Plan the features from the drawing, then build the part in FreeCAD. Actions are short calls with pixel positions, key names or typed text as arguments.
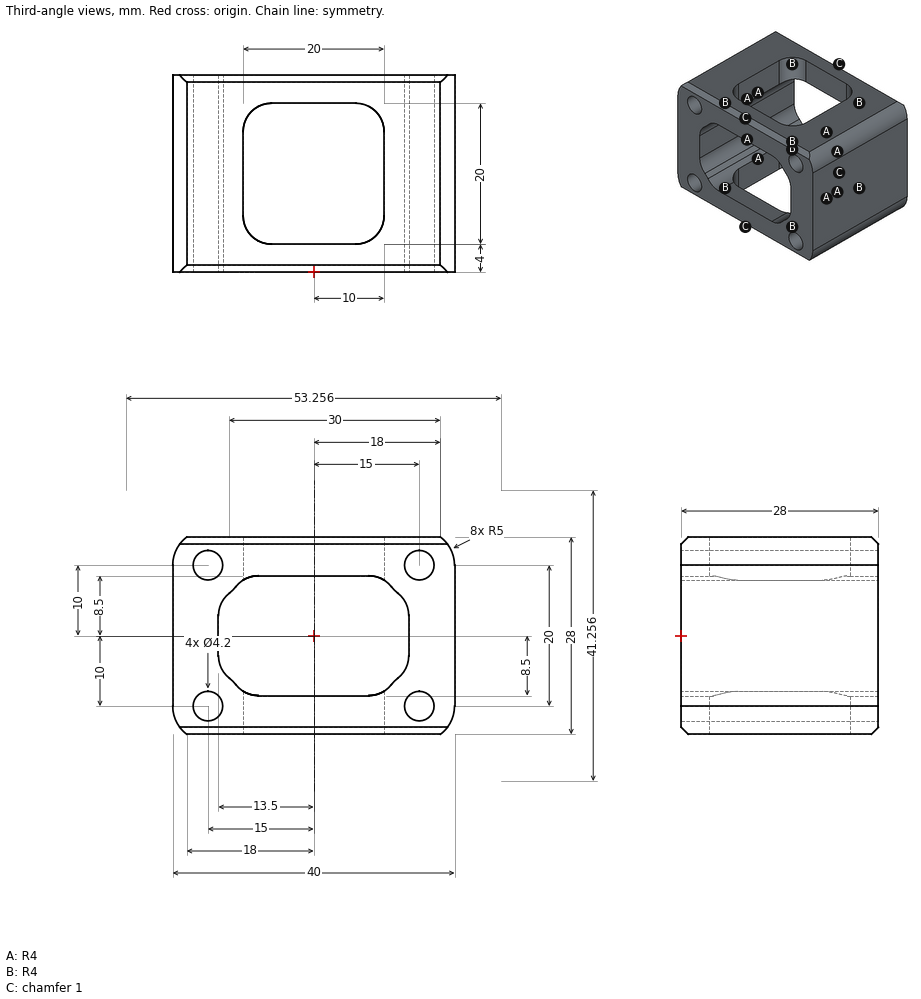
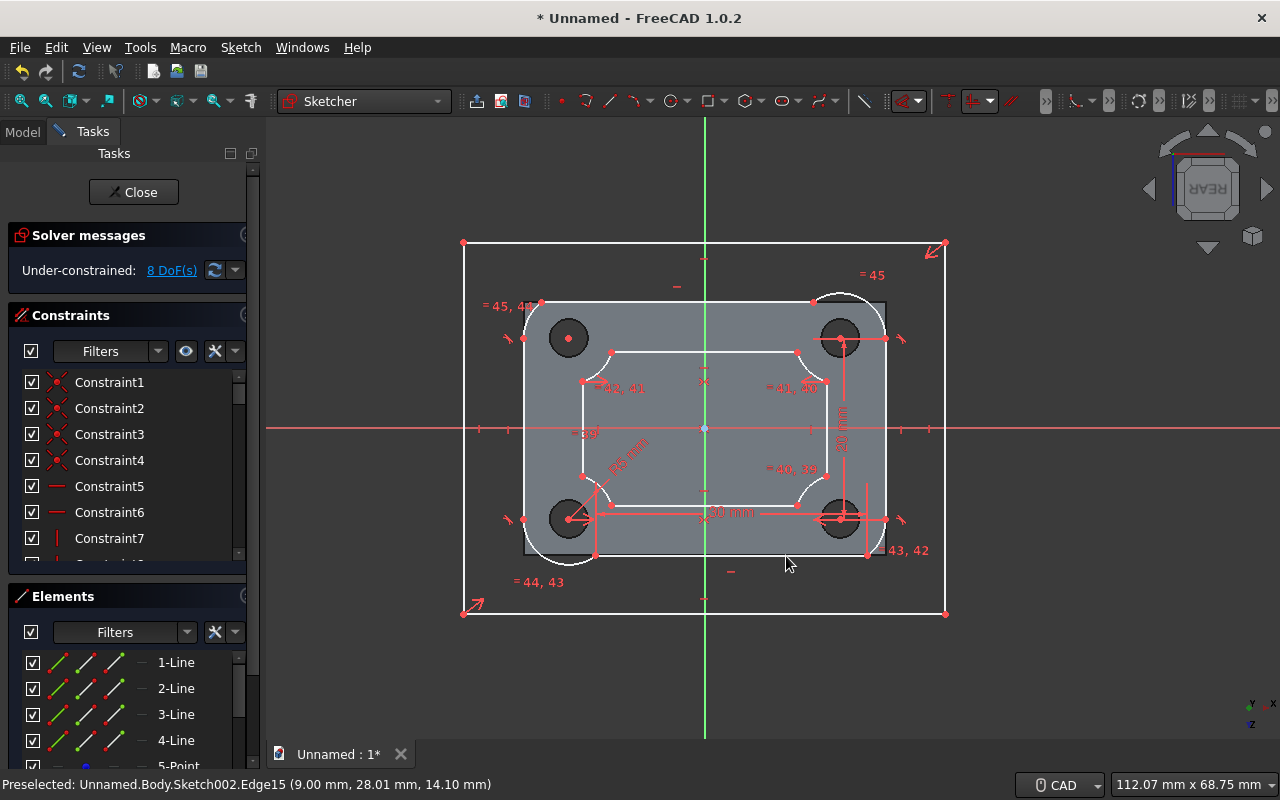
click(886, 339)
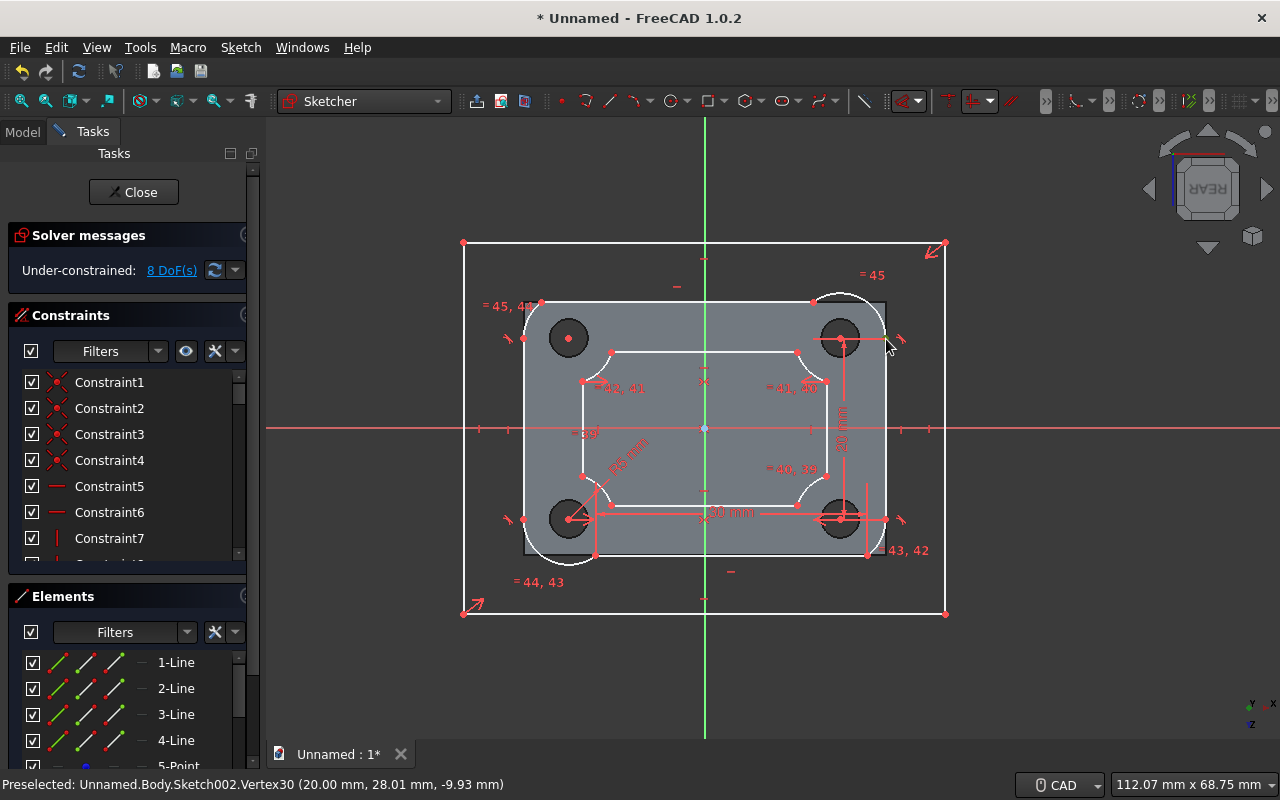
key(i)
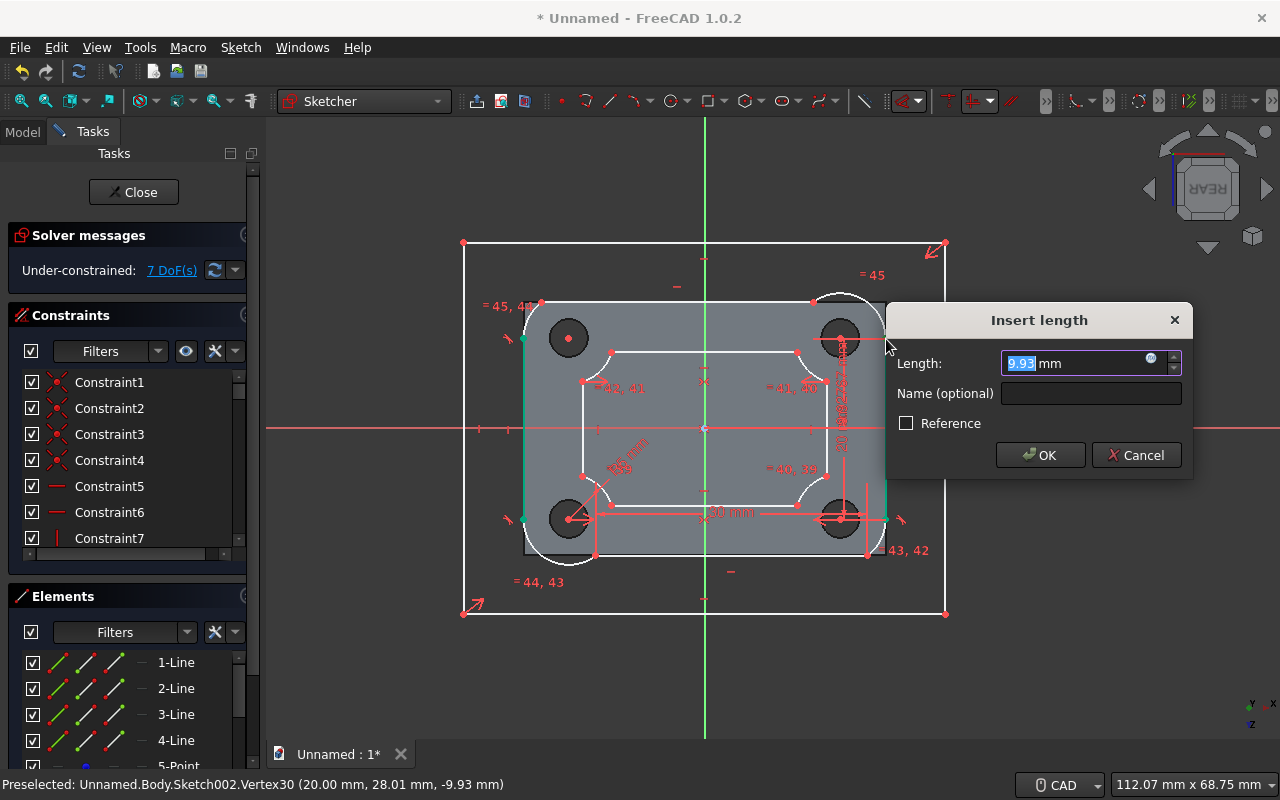
text(10)
key(Return)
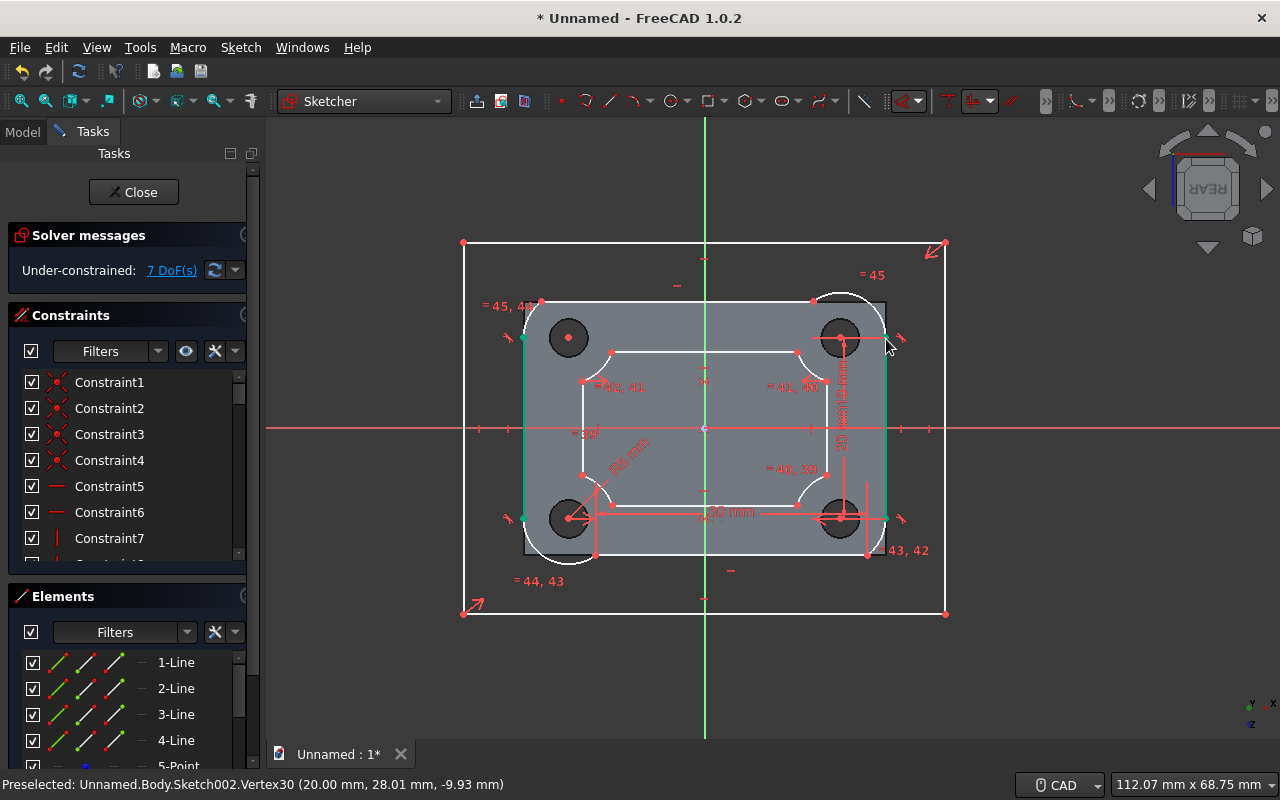
click(867, 555)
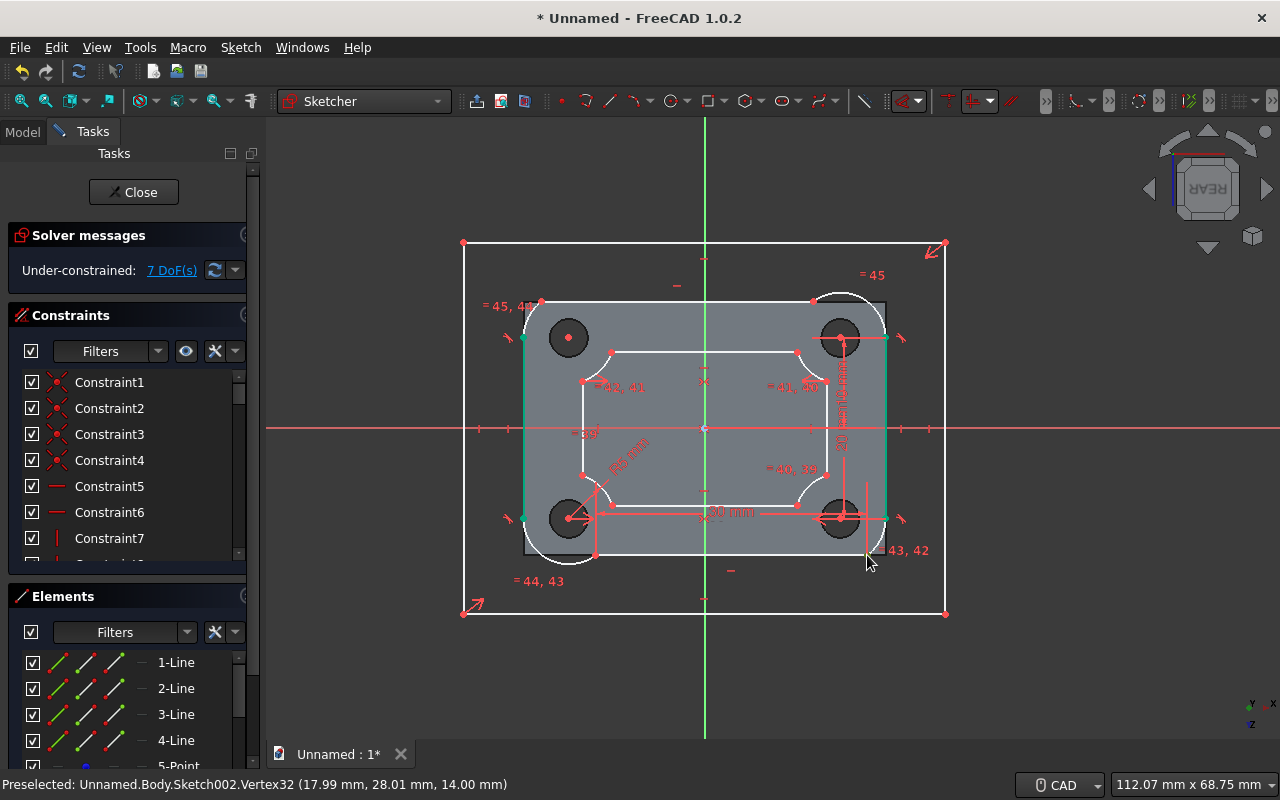
click(920, 102)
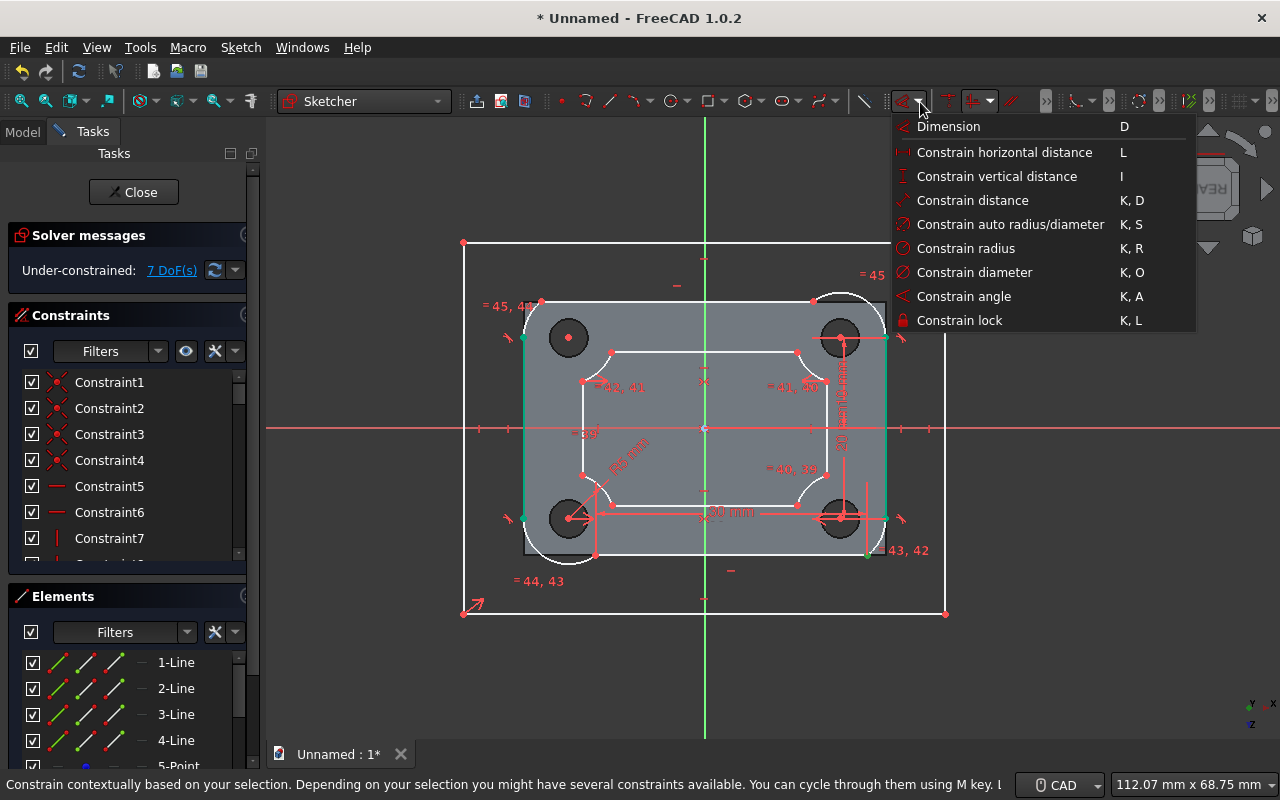
click(1044, 152)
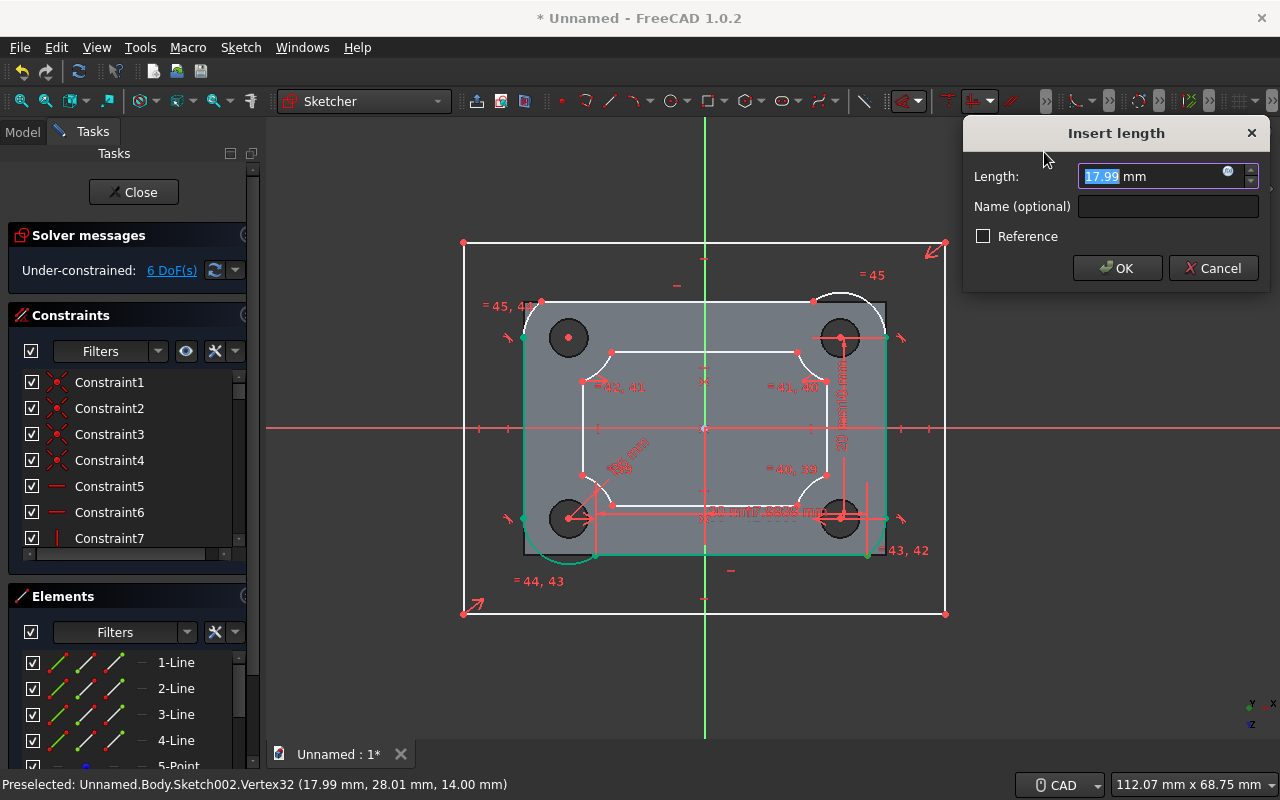
text(18)
key(Return)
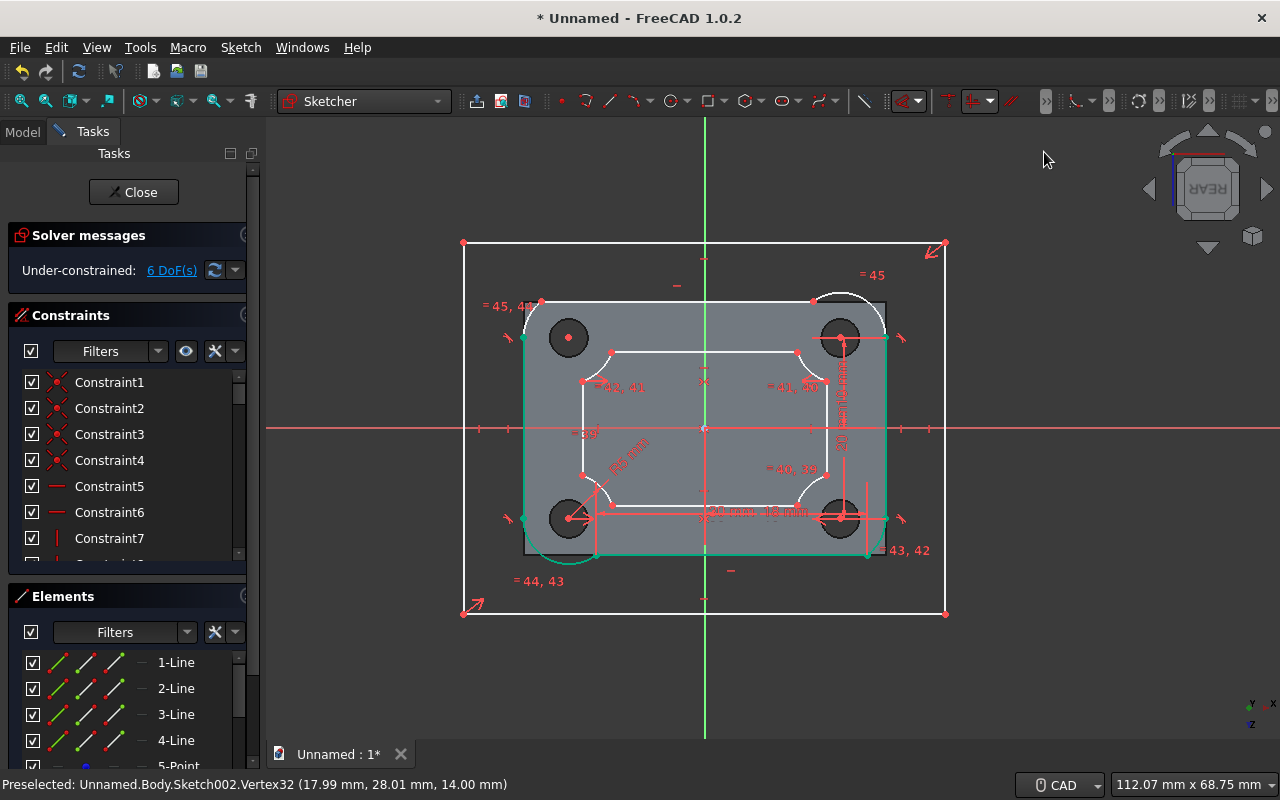
click(542, 302)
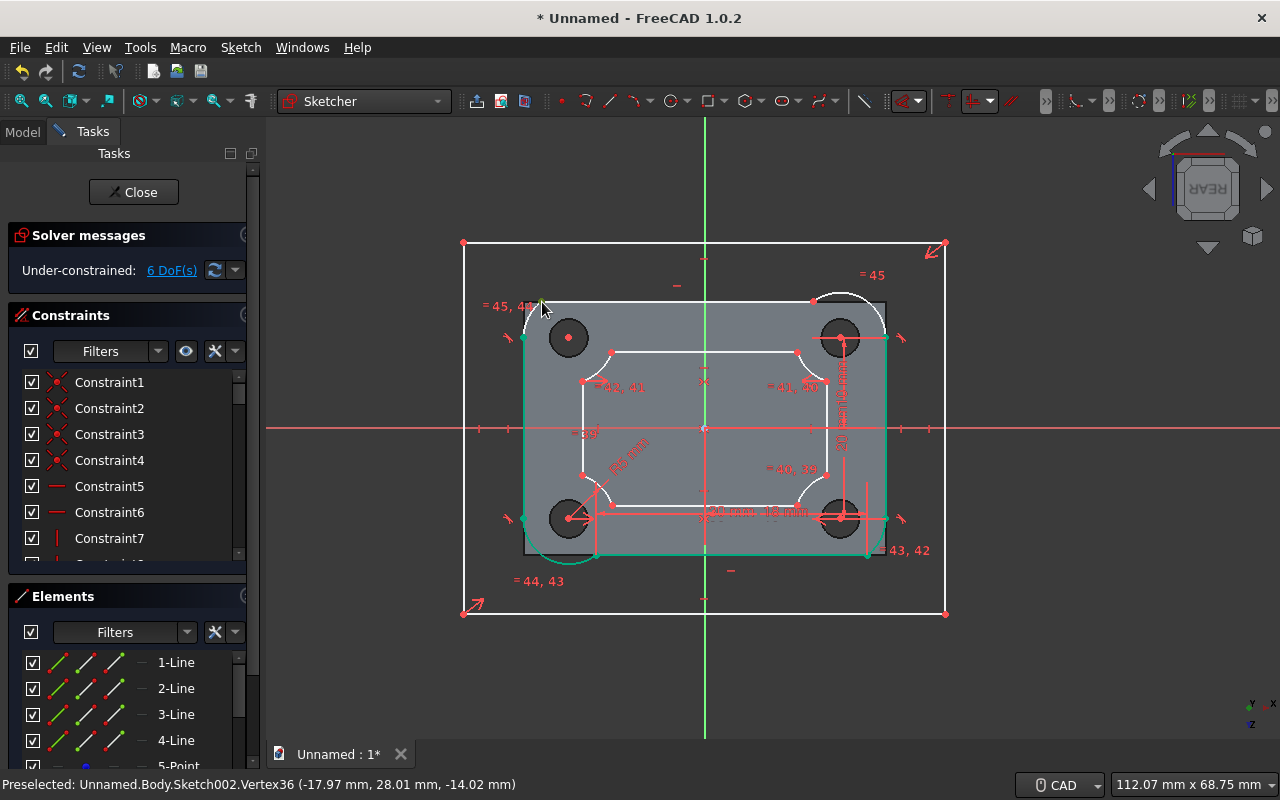
key(l)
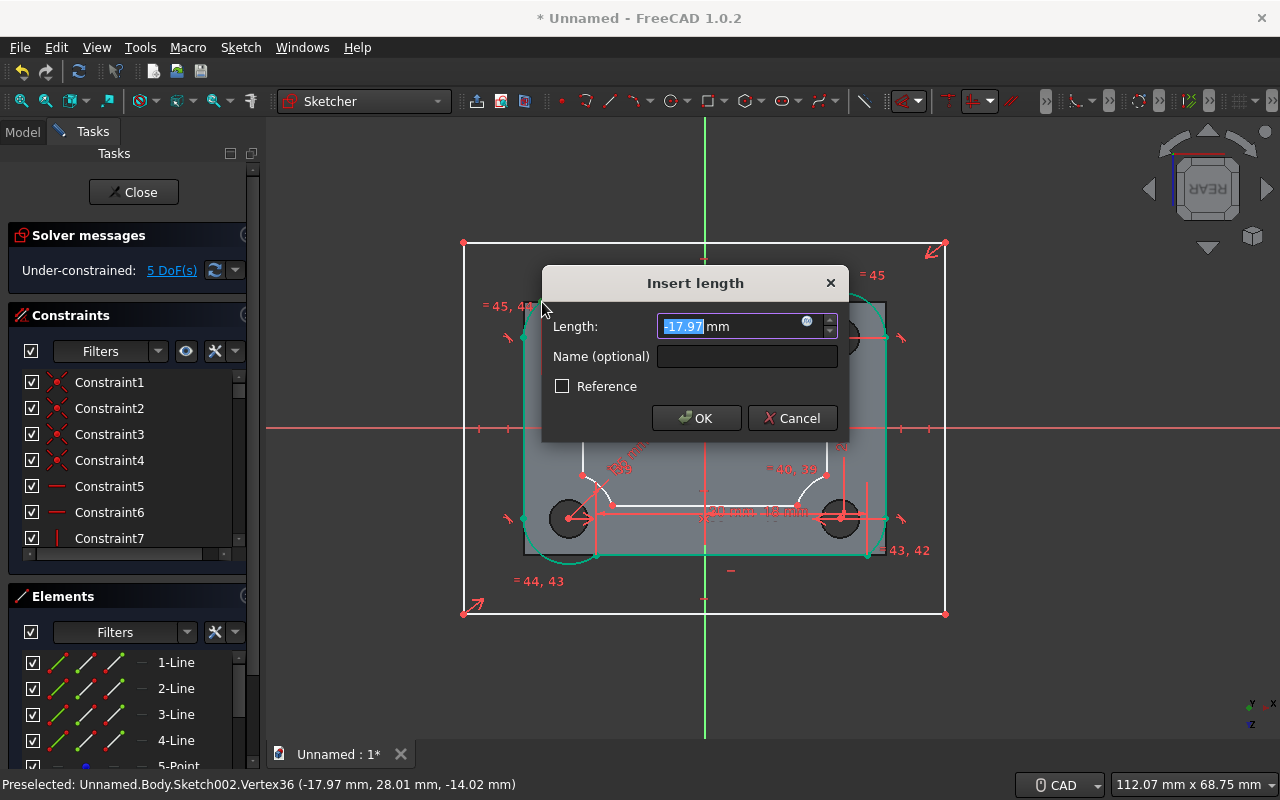
text(-18)
key(Return)